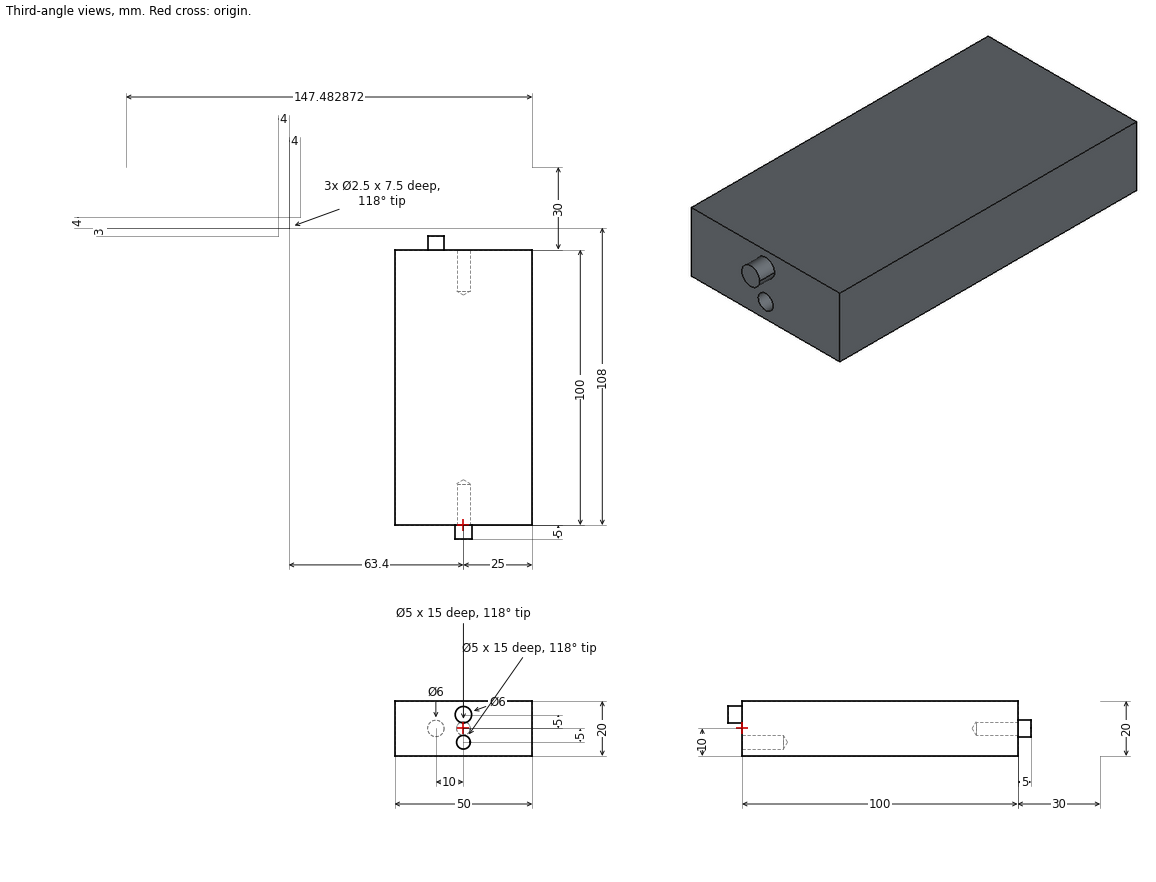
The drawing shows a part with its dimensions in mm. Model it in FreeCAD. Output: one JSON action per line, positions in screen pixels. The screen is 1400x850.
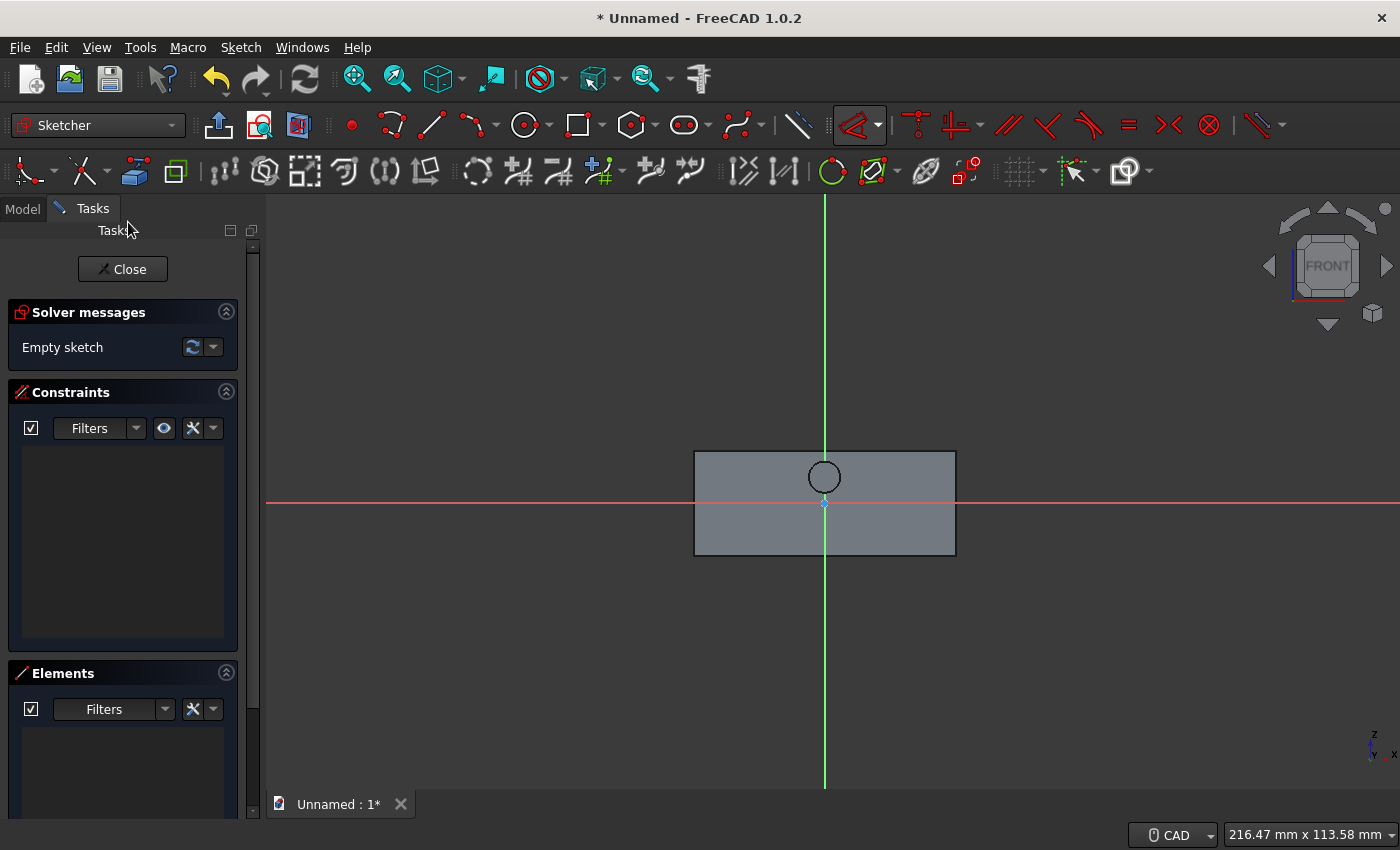
{"action": "key", "text": "q s"}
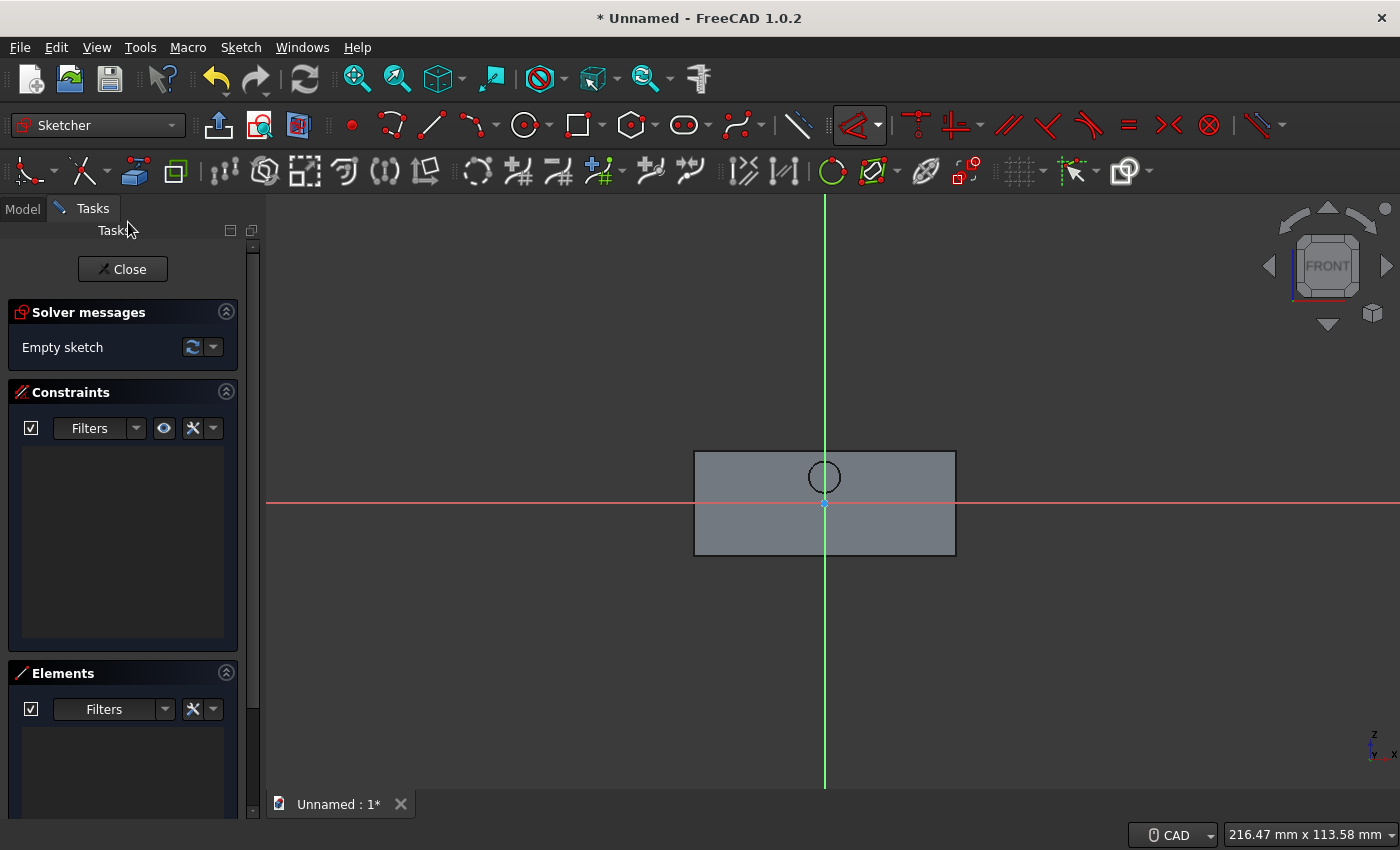
{"action": "scroll", "coordinate": [832, 527], "scroll_direction": "up", "scroll_amount": 11}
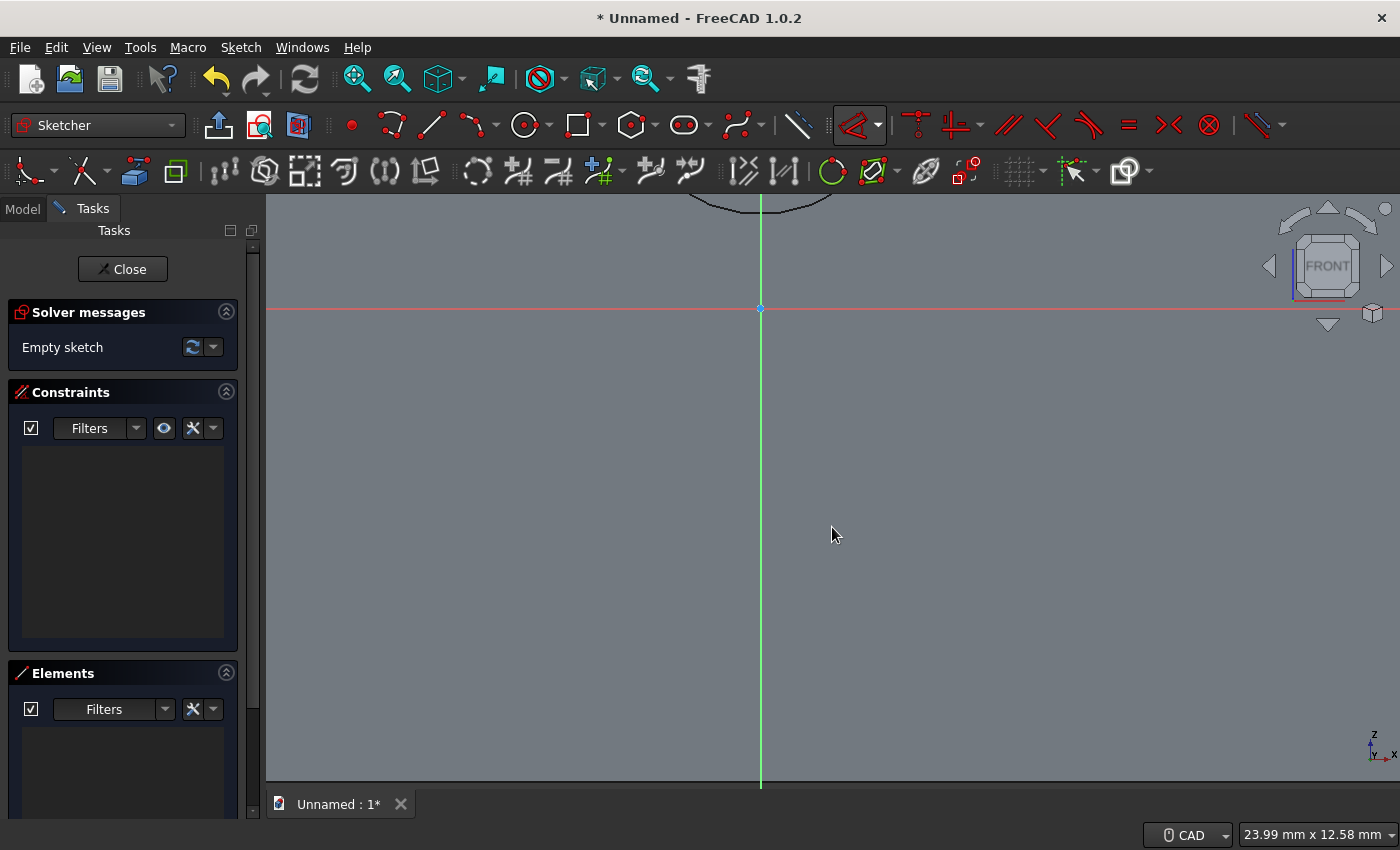
{"action": "key", "text": "g c"}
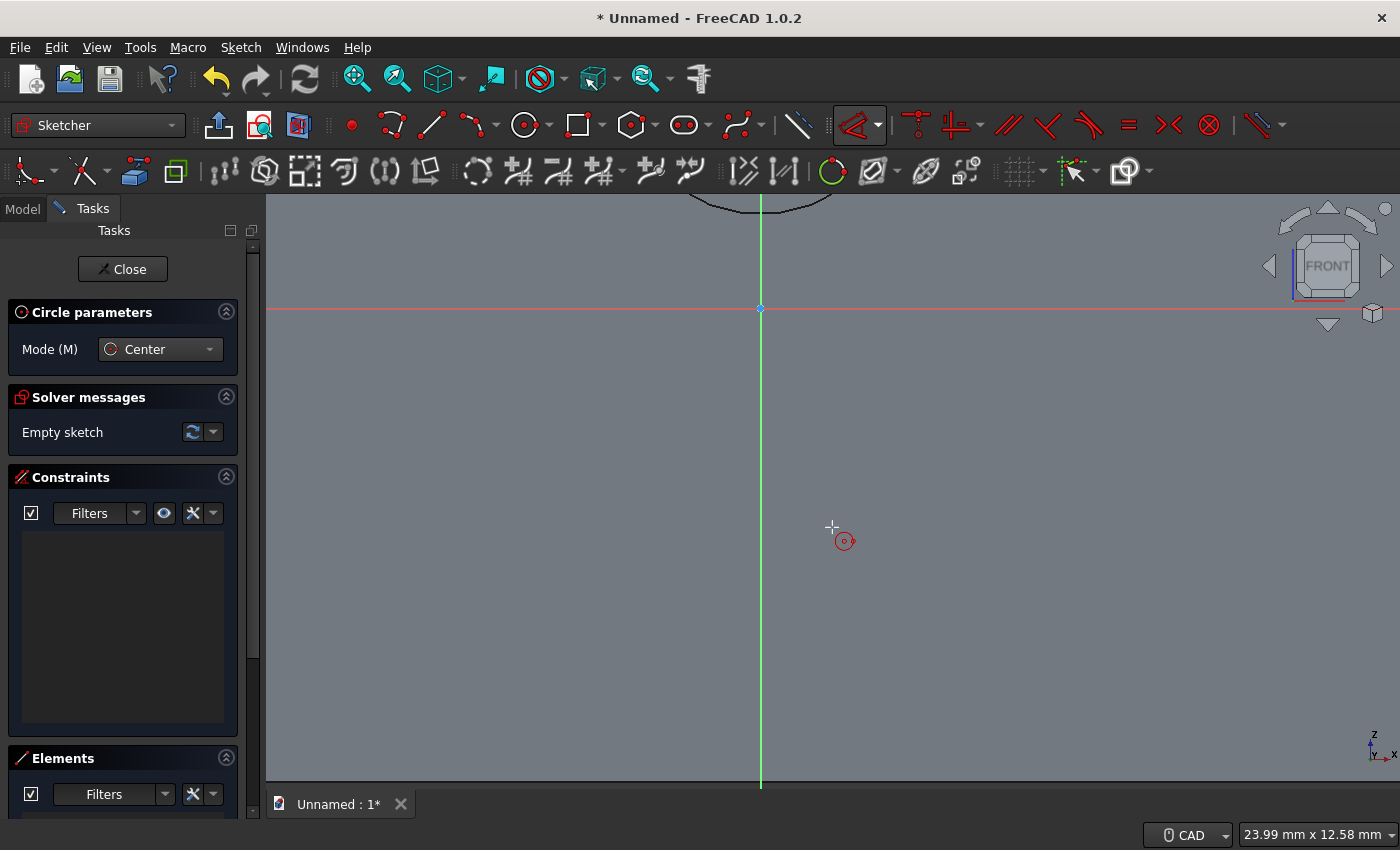
{"action": "left_click", "coordinate": [761, 545]}
{"action": "left_click", "coordinate": [844, 462]}
{"action": "key", "text": "Escape"}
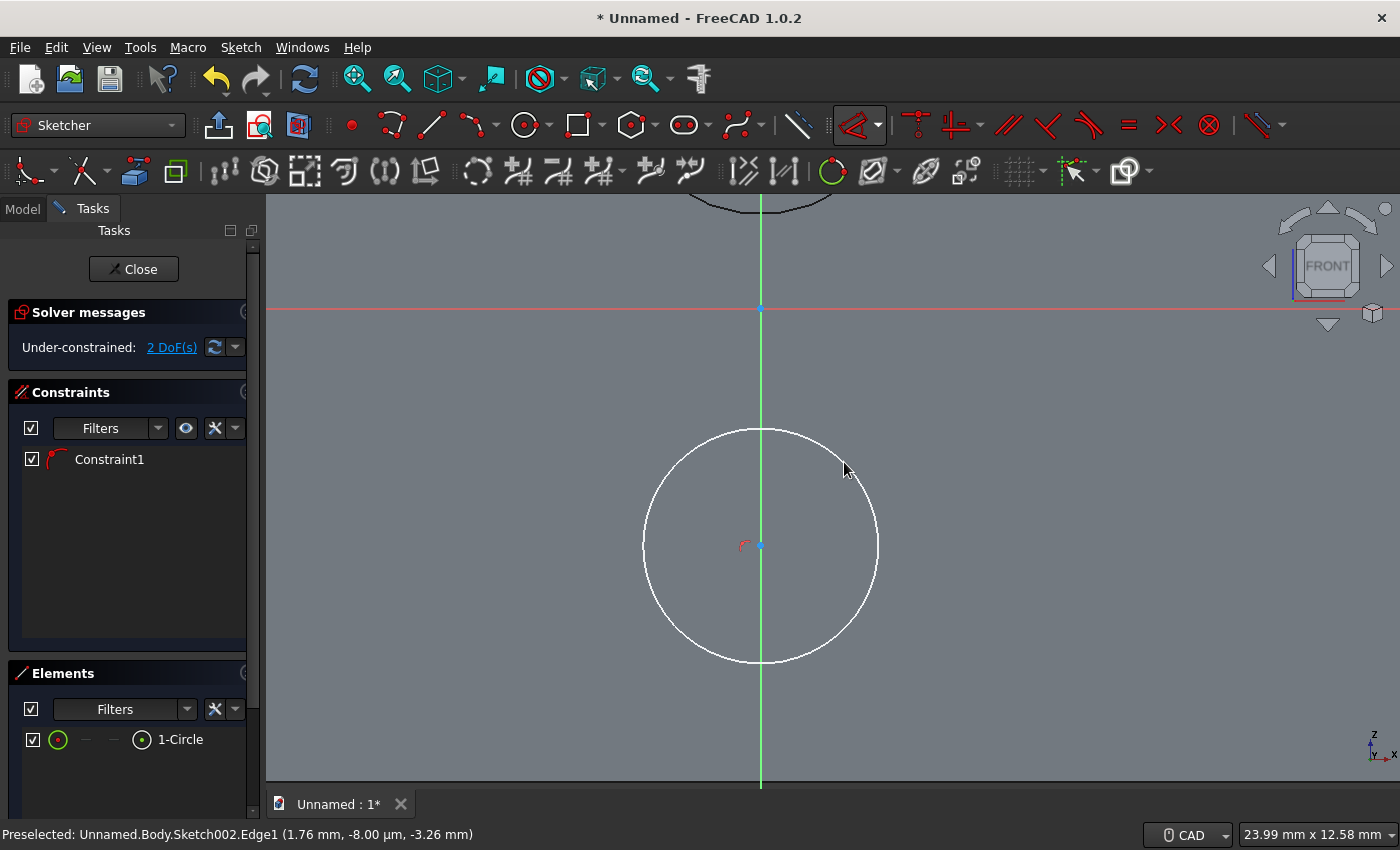
{"action": "left_click", "coordinate": [844, 463]}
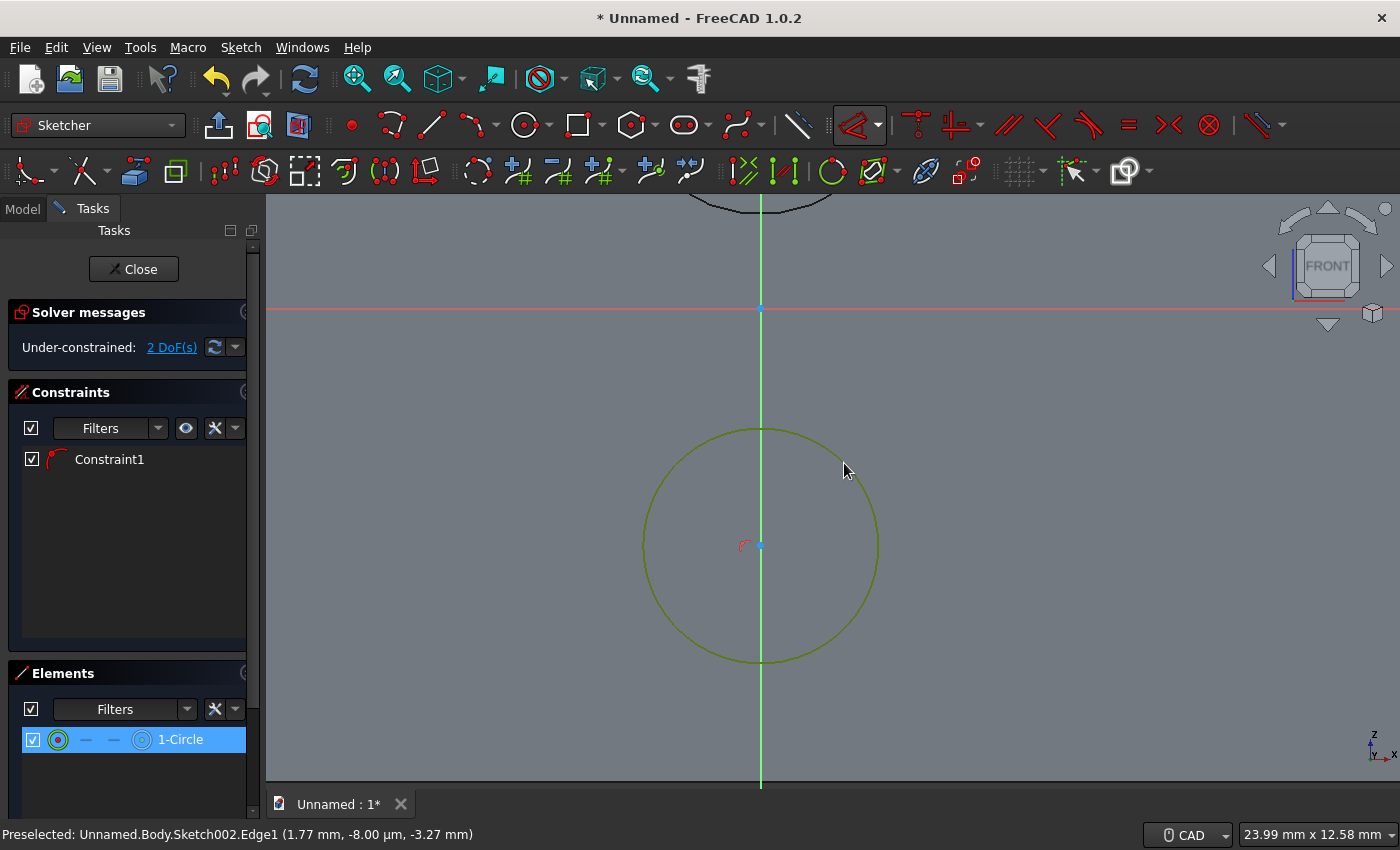
{"action": "key", "text": "k o"}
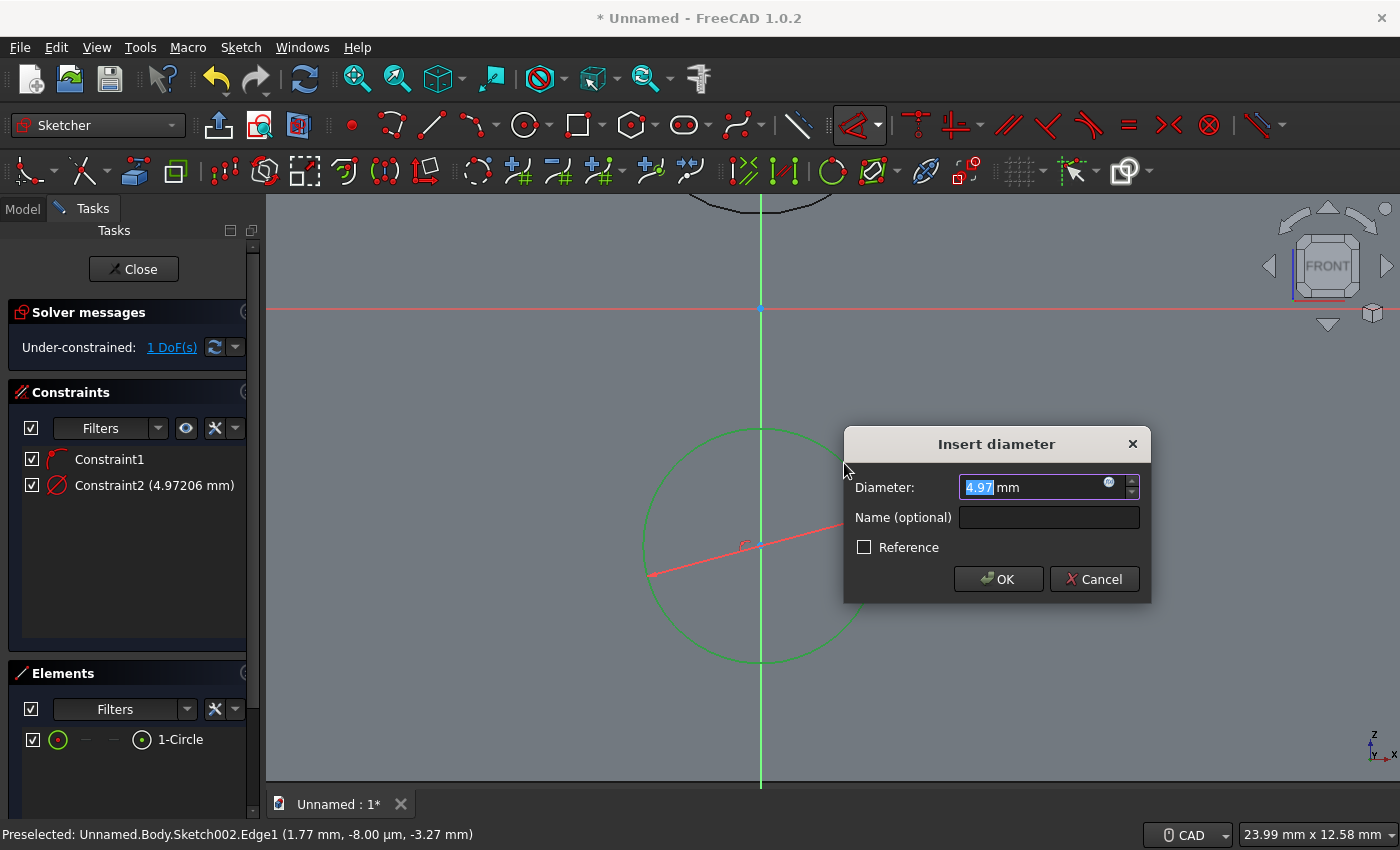
{"action": "type", "text": "5"}
{"action": "key", "text": "Return"}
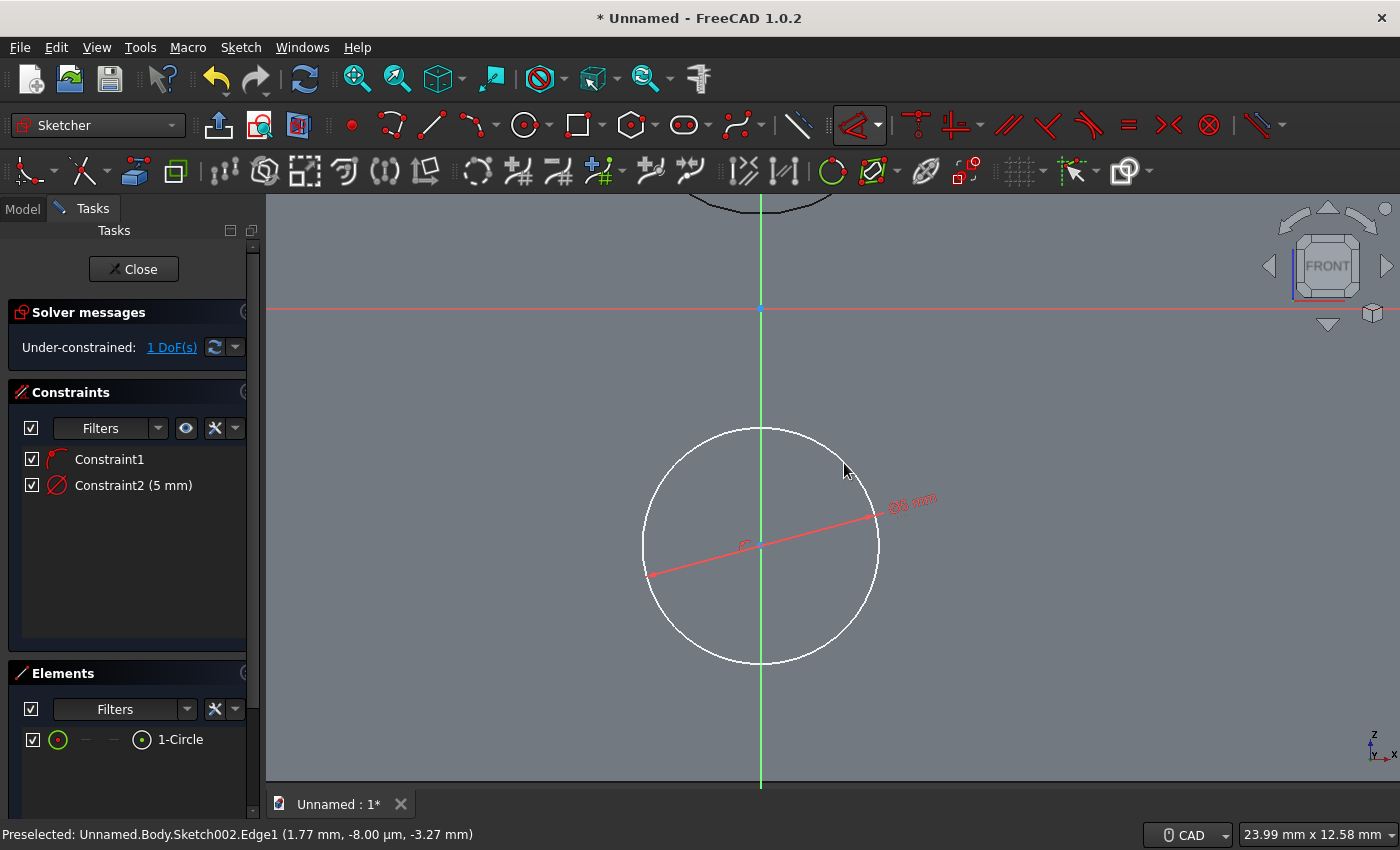
{"action": "left_click", "coordinate": [761, 546]}